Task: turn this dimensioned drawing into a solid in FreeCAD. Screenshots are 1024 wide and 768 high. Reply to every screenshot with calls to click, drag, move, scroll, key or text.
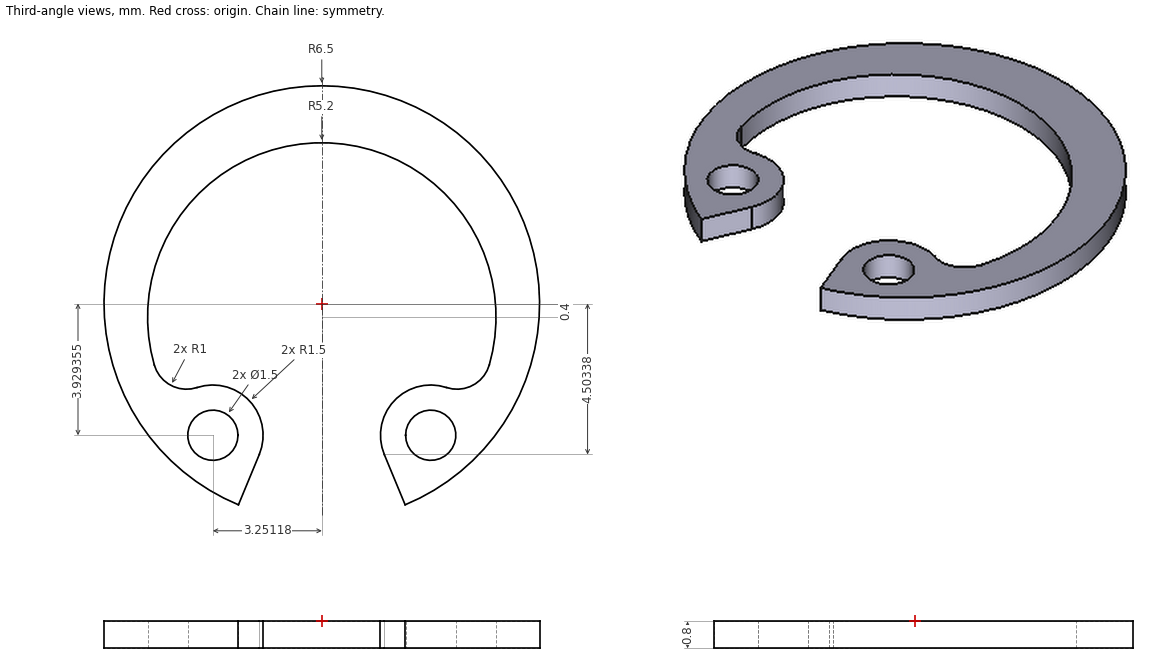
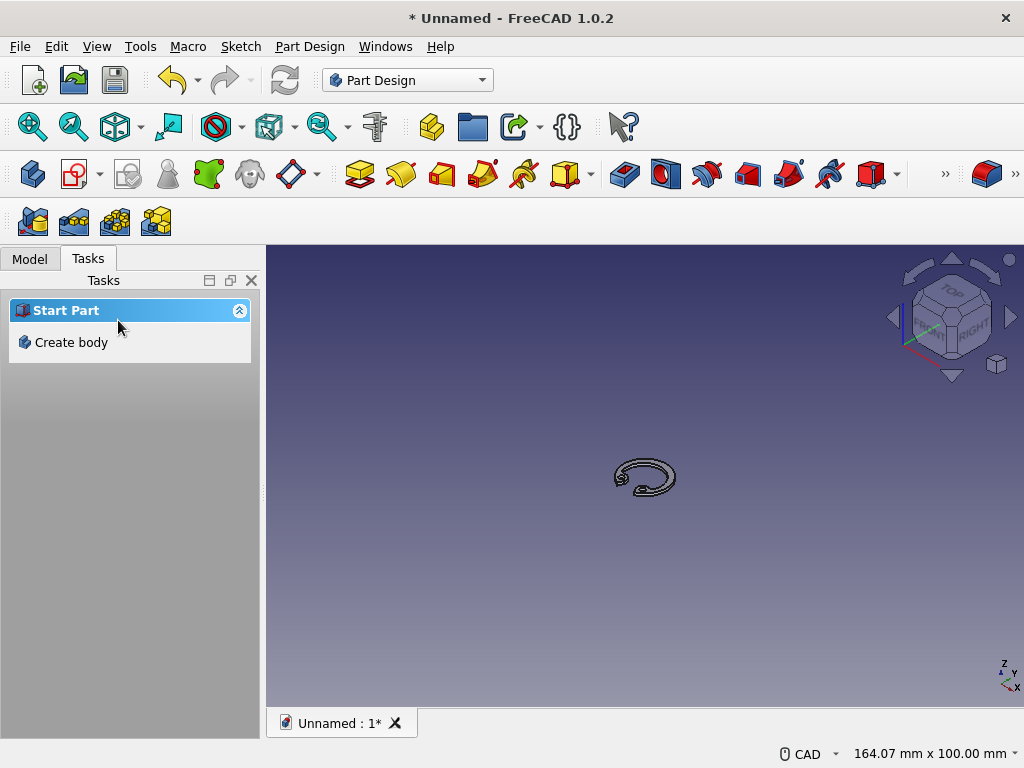
click(33, 128)